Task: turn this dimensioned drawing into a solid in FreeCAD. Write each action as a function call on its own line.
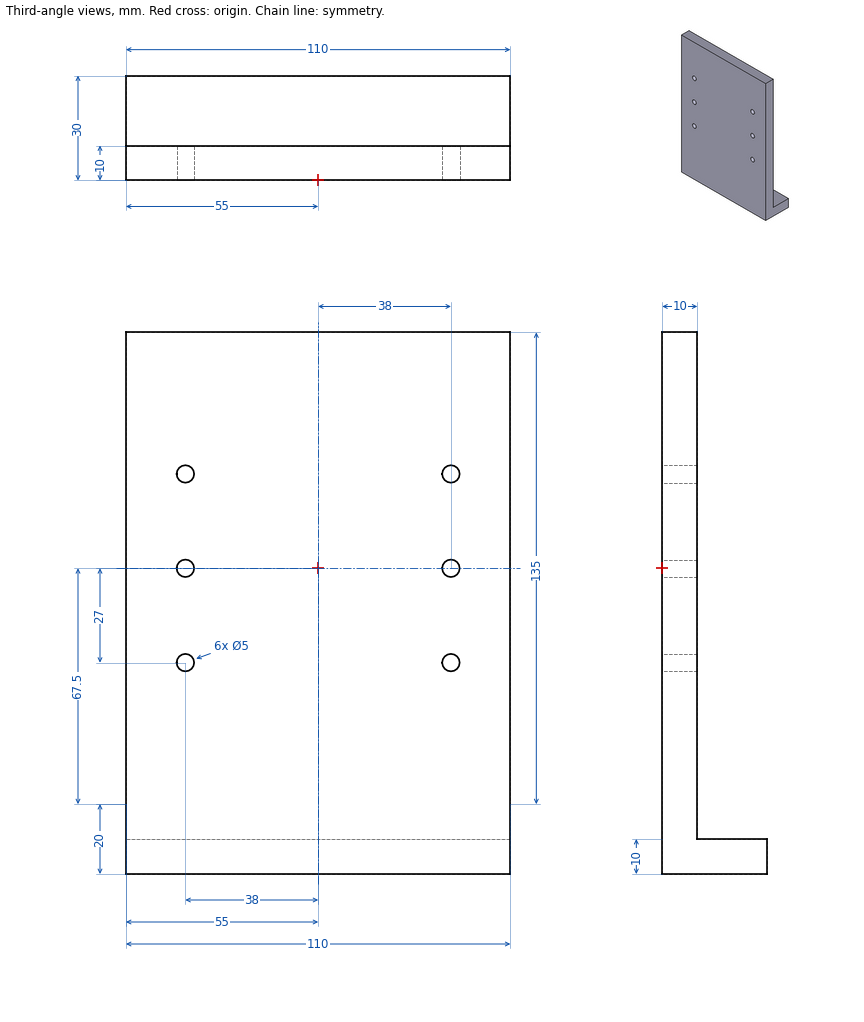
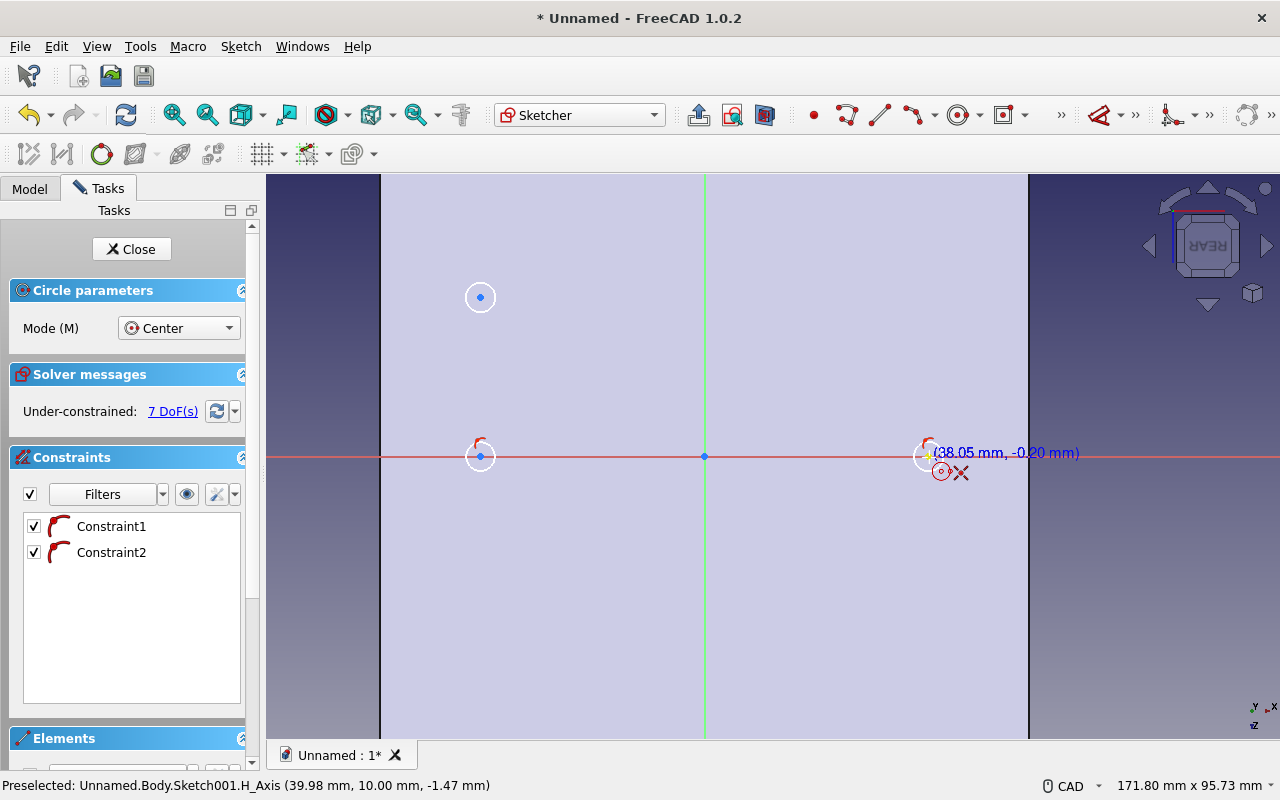
scroll(480, 616, up, 3)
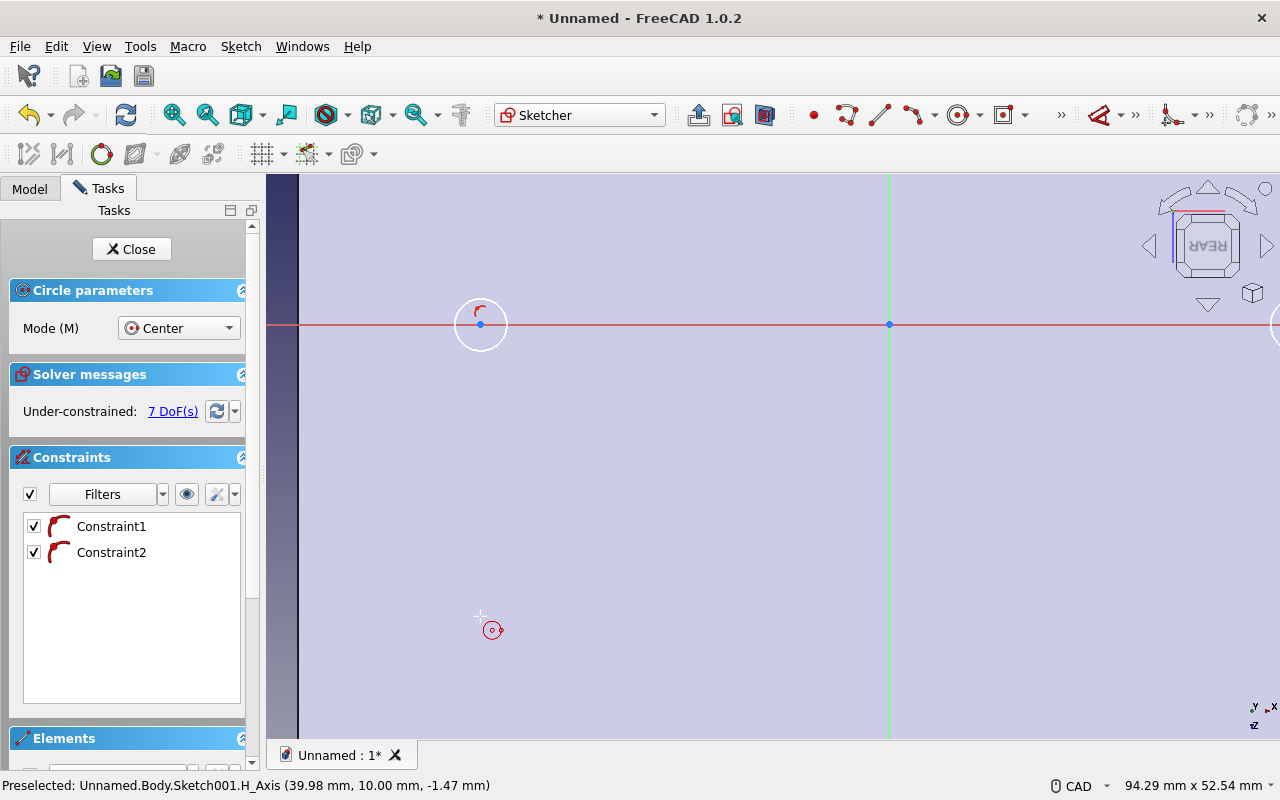
click(481, 615)
click(500, 596)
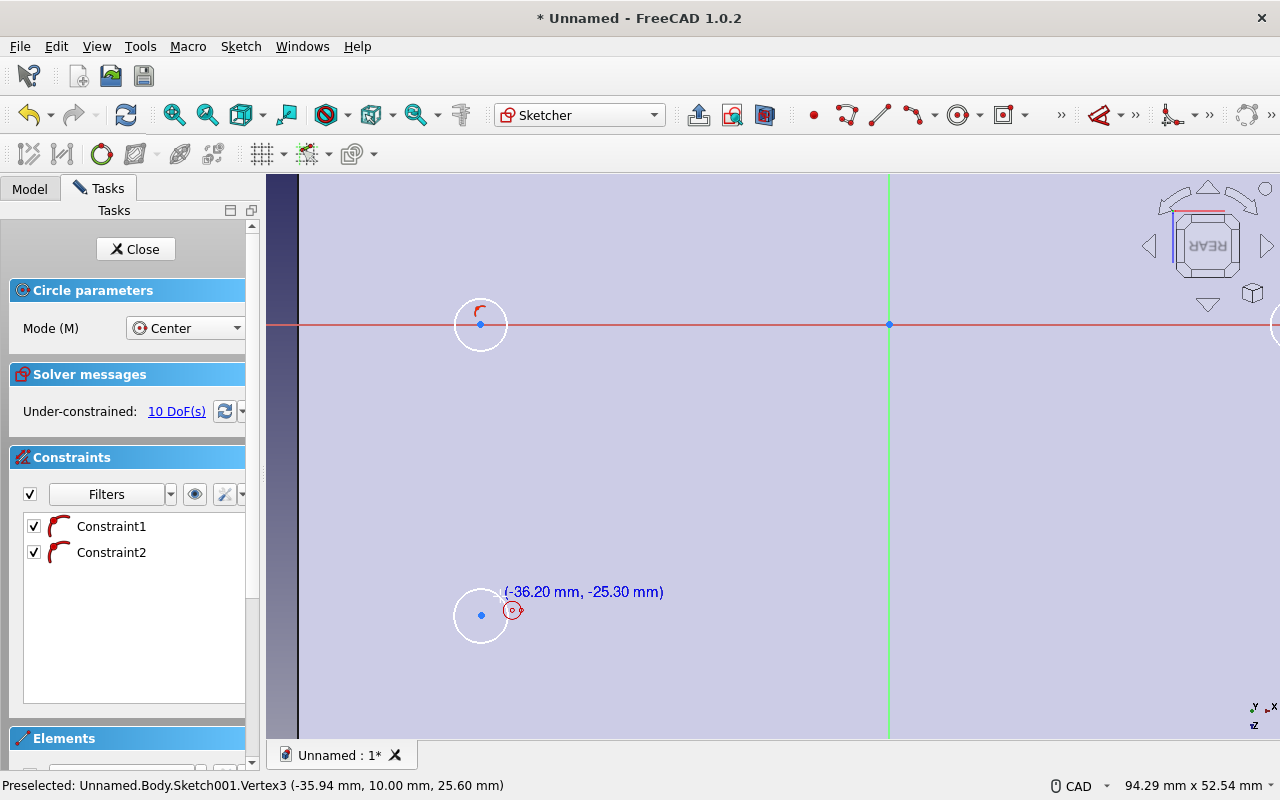
scroll(480, 617, down, 3)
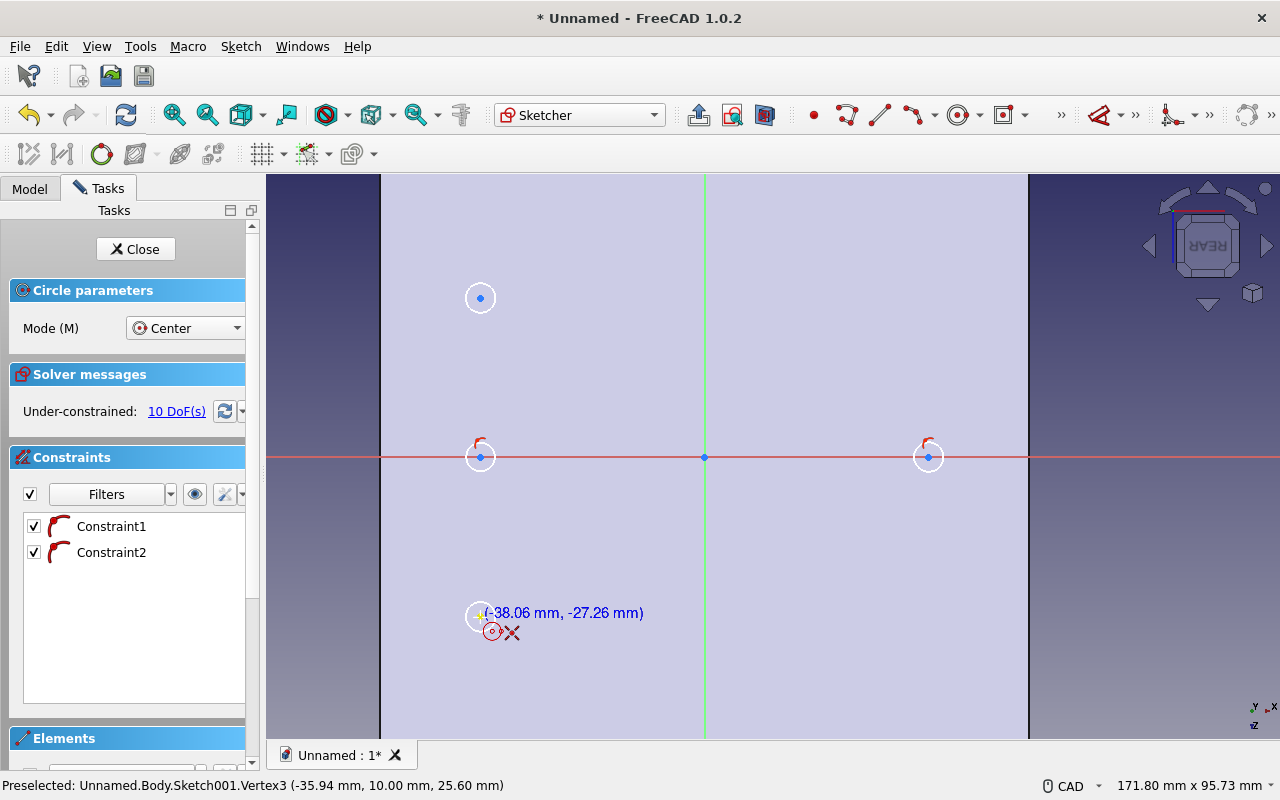
scroll(929, 616, up, 3)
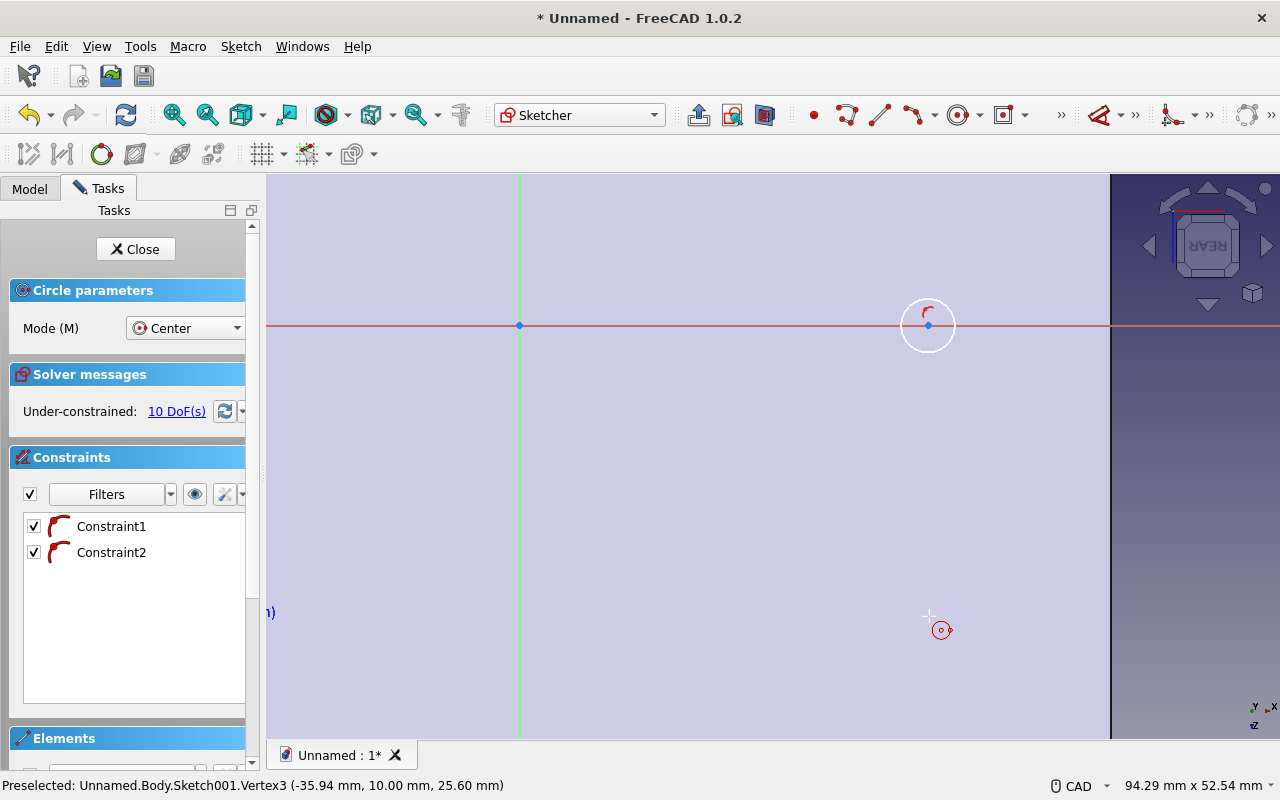
click(928, 616)
click(948, 597)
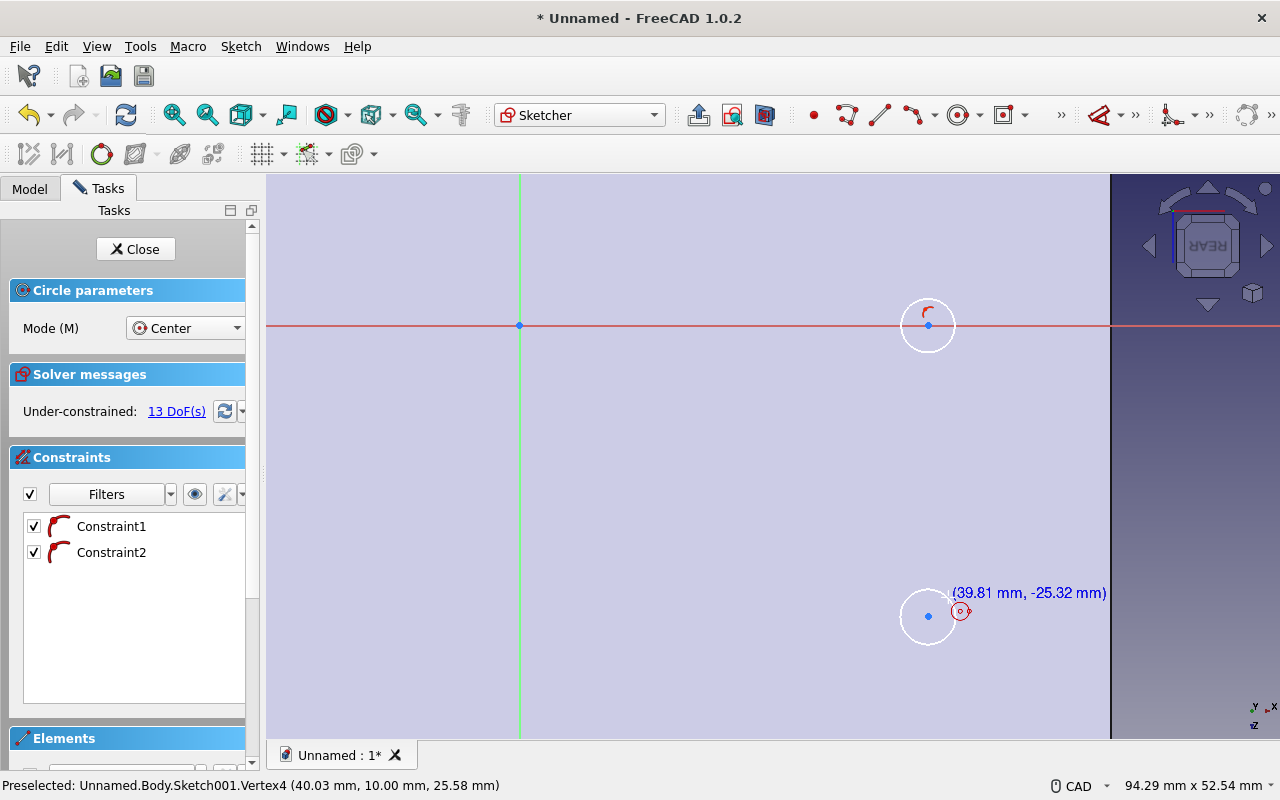
scroll(929, 616, down, 3)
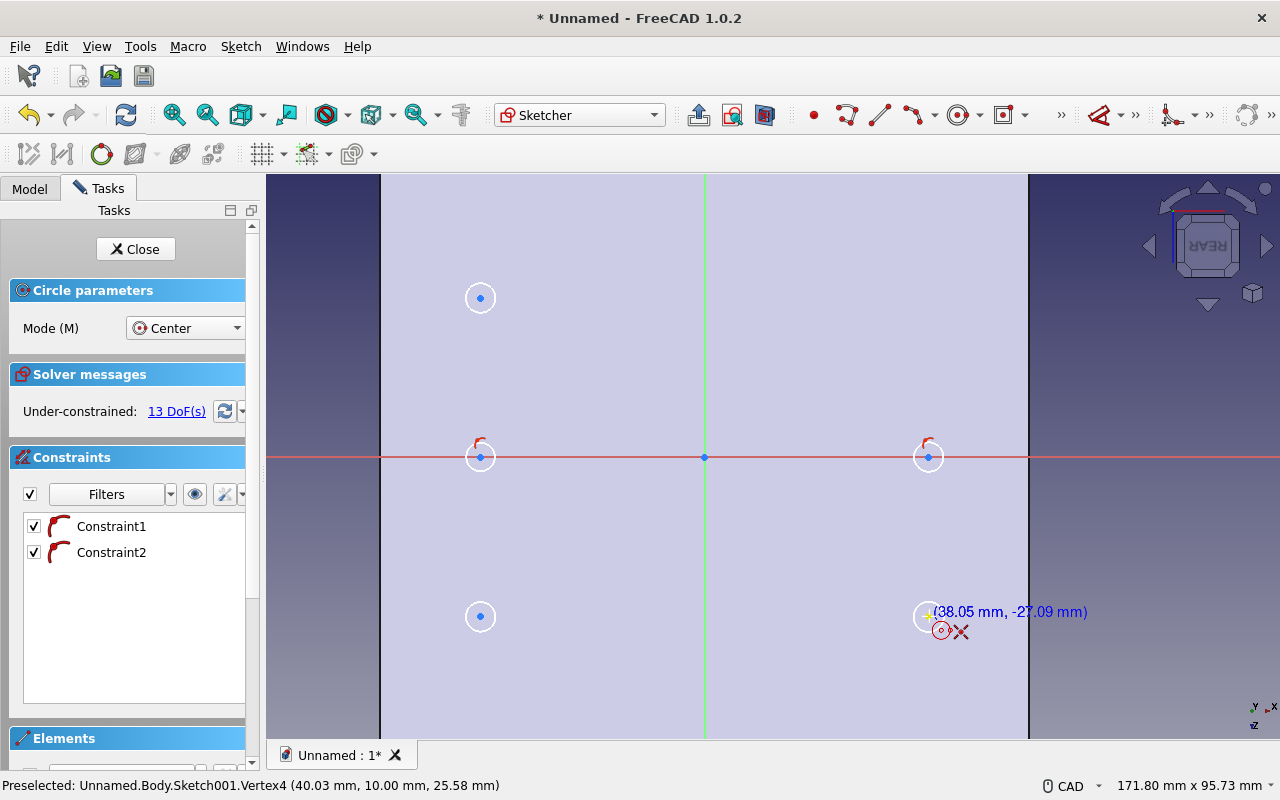
scroll(929, 298, up, 3)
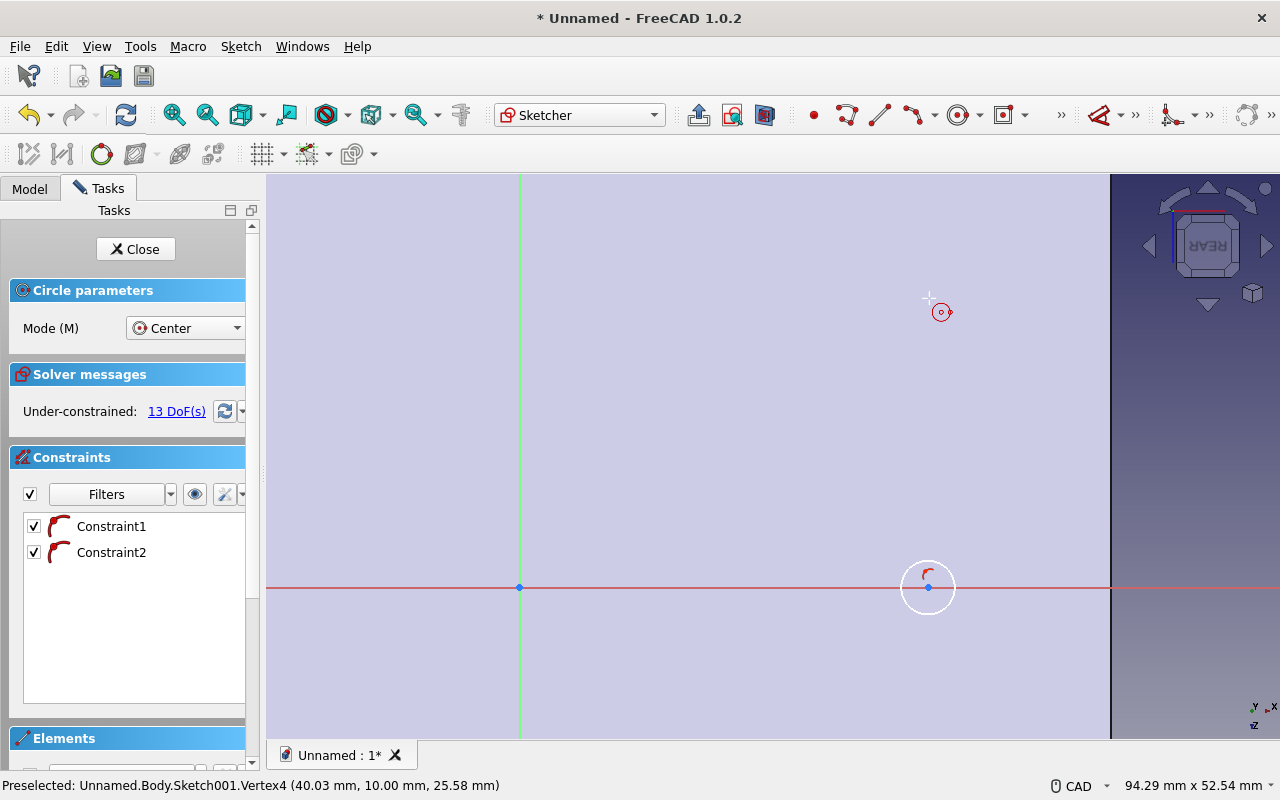
click(928, 297)
click(948, 278)
key(Escape)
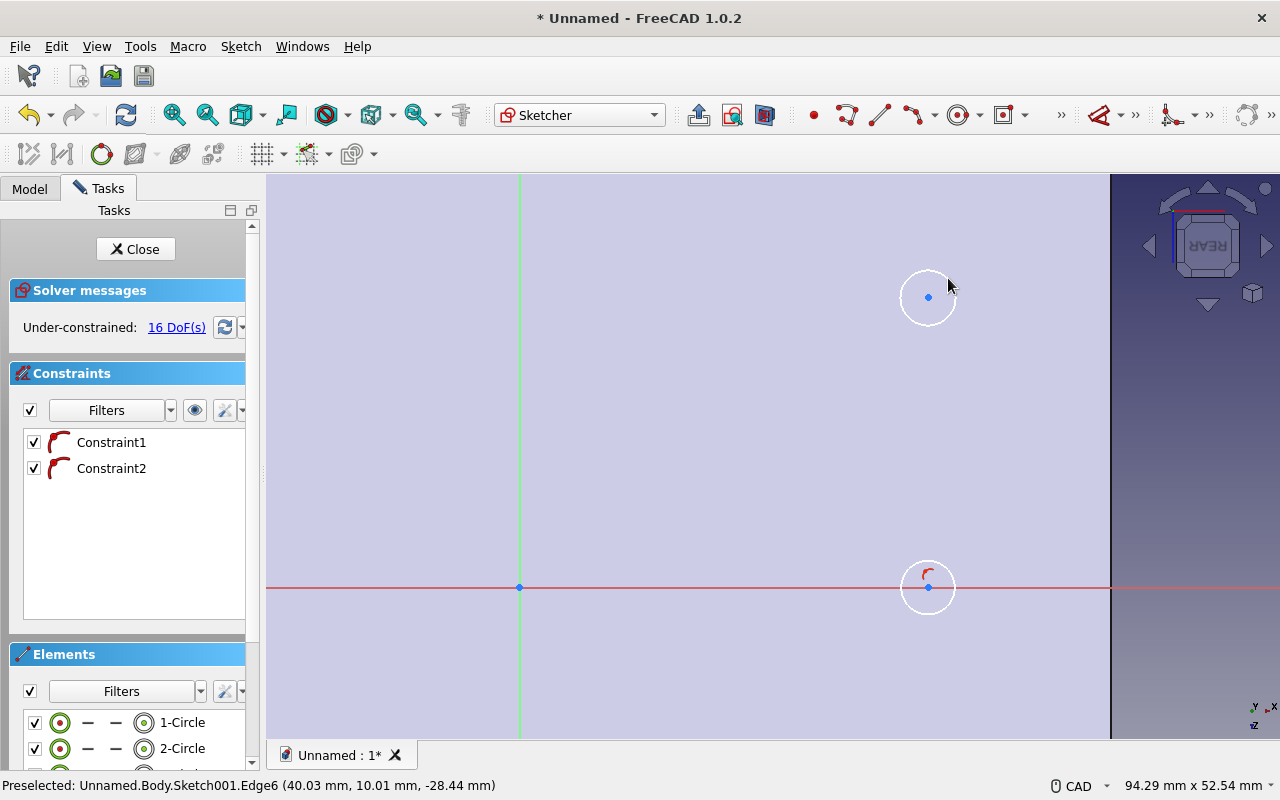
scroll(929, 297, down, 3)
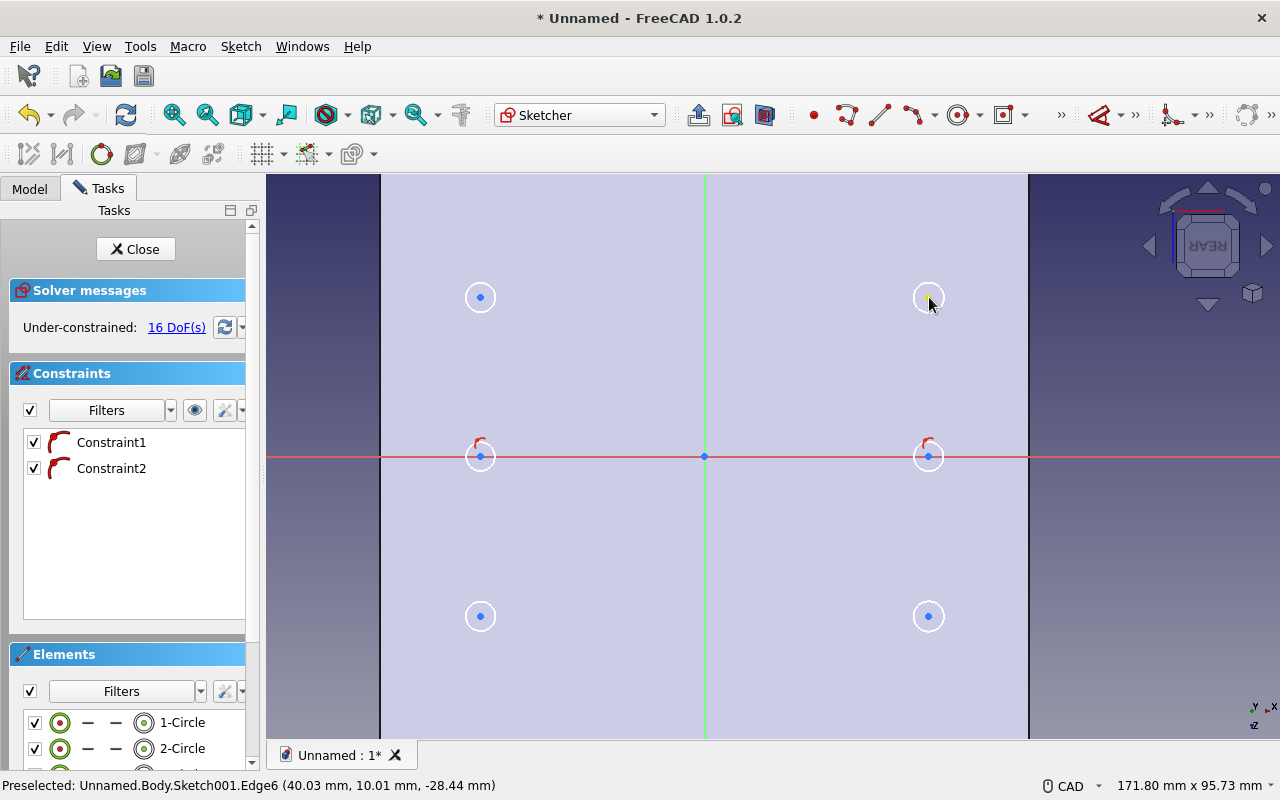
click(491, 287)